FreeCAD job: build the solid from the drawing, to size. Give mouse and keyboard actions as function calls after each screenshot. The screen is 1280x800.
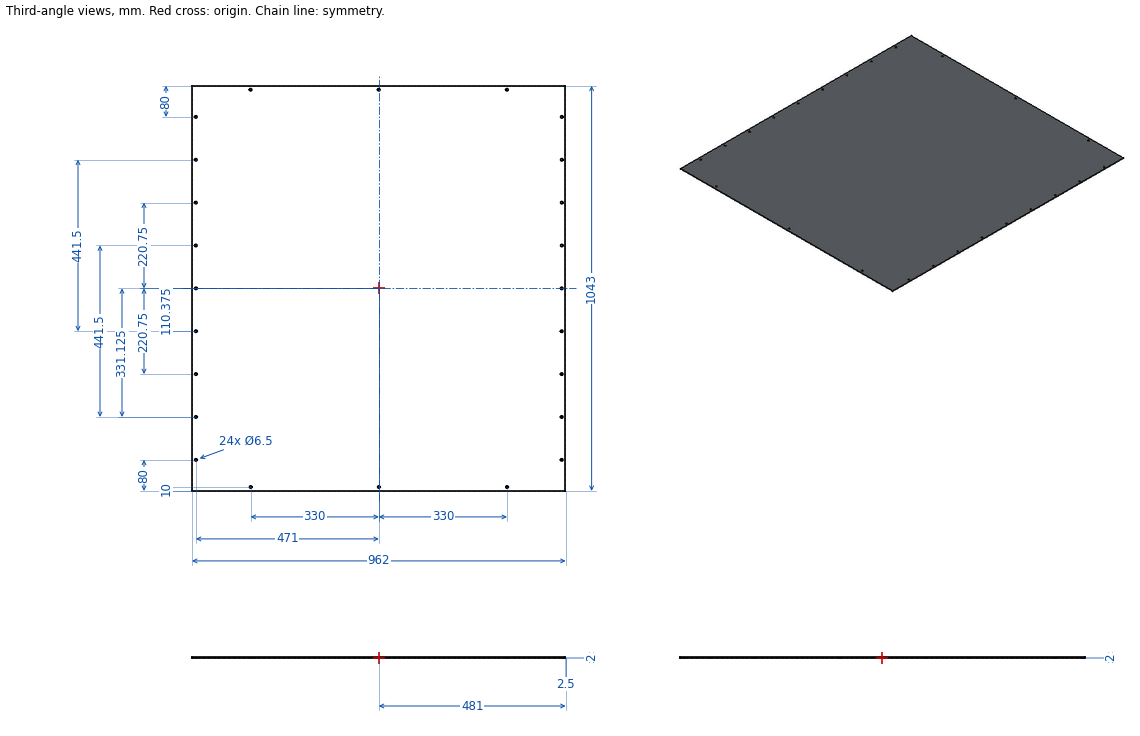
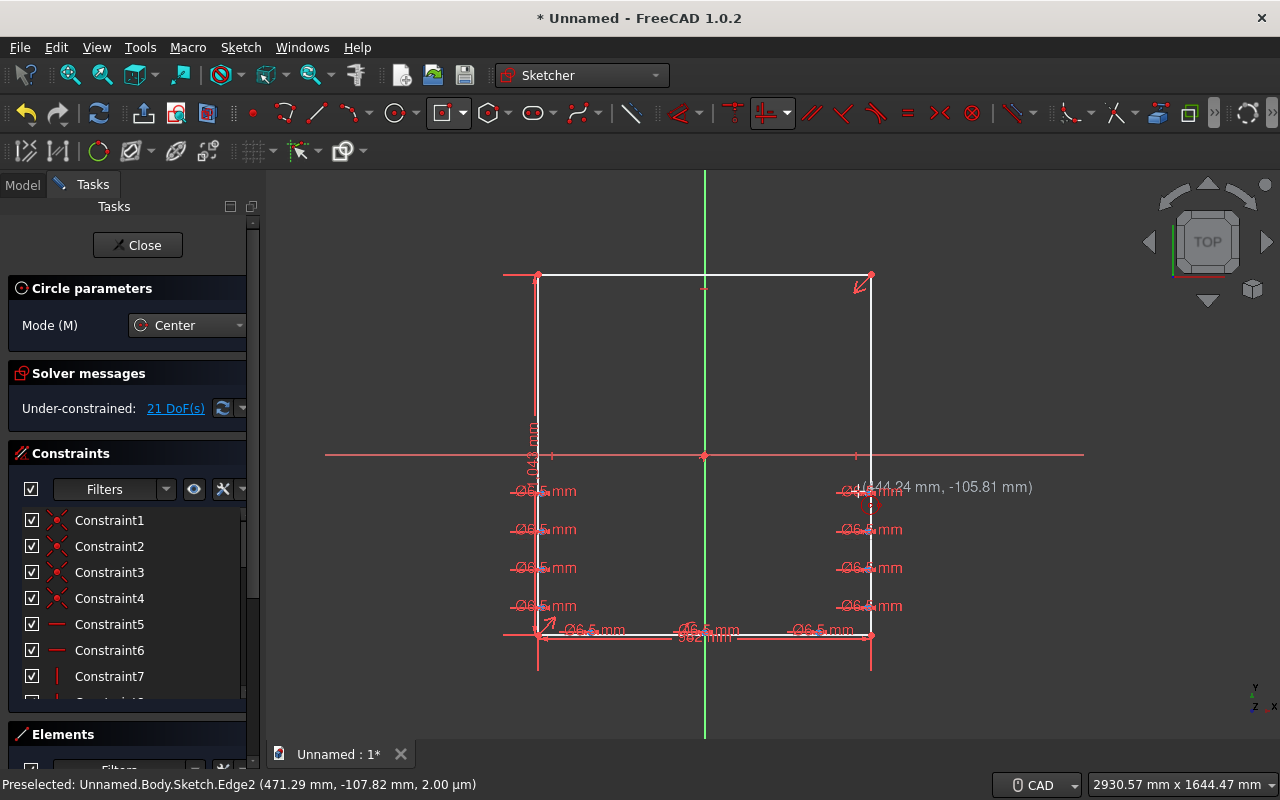
scroll(542, 455, up, 16)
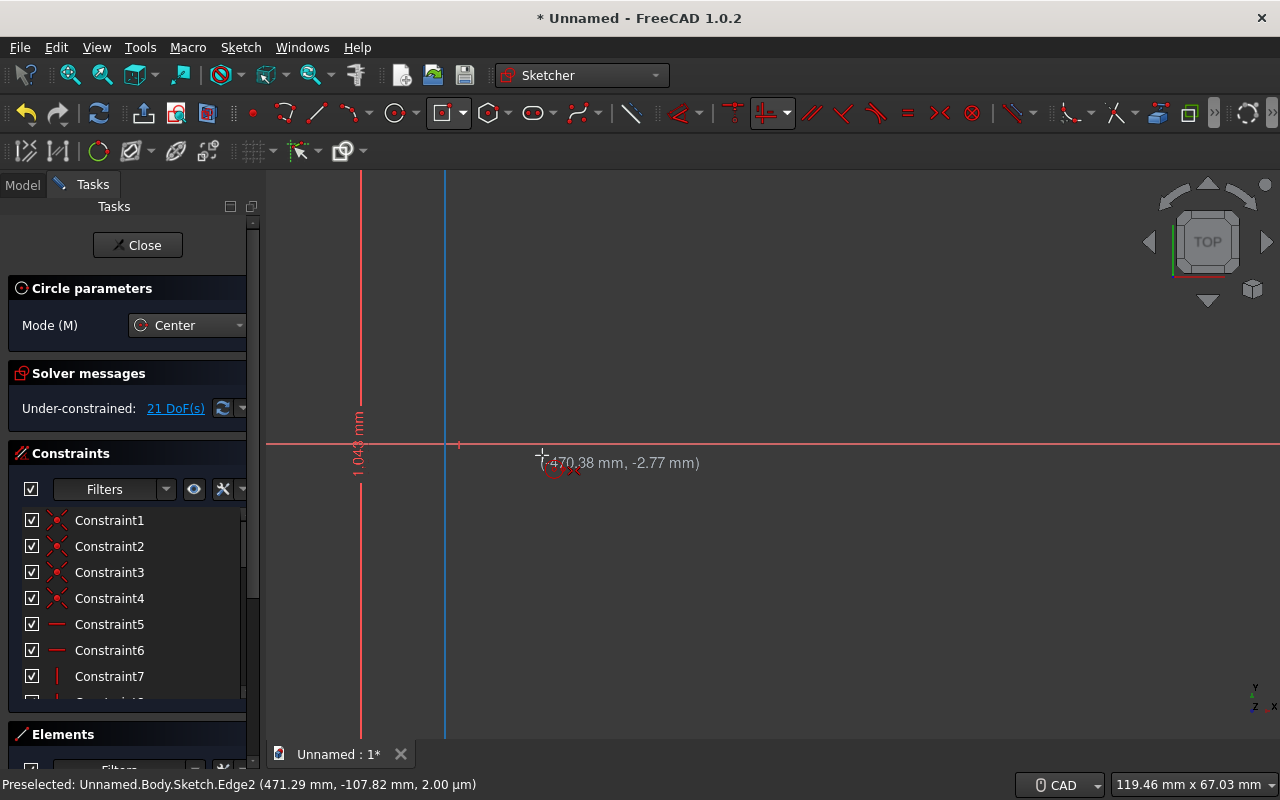
scroll(504, 455, down, 15)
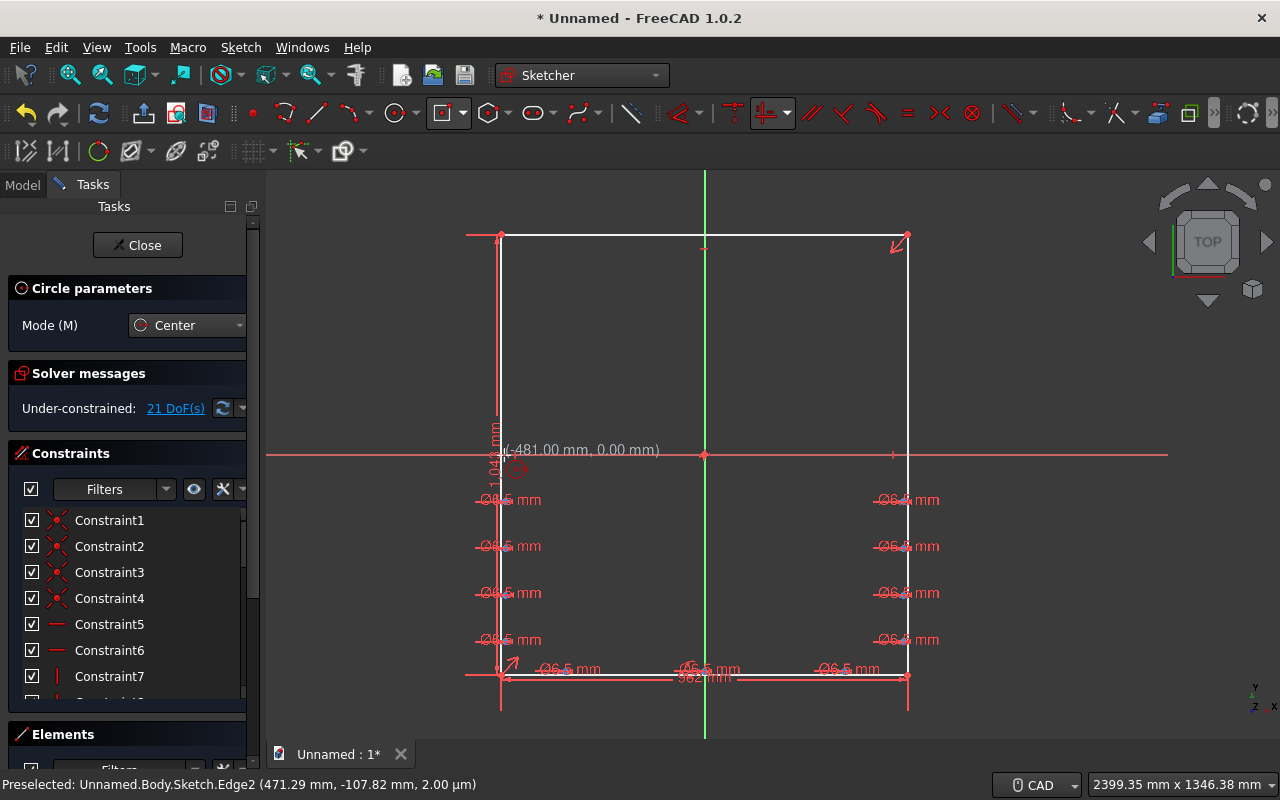
scroll(506, 455, up, 7)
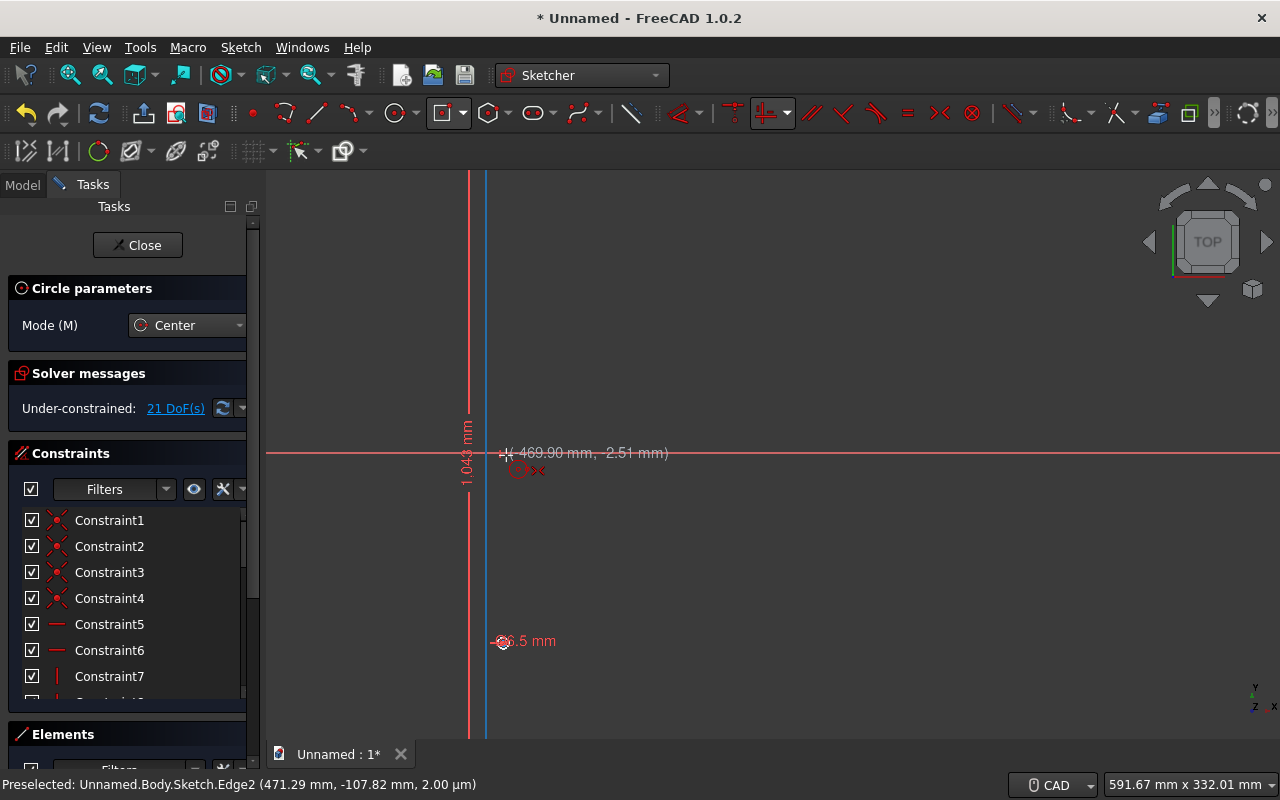
click(503, 453)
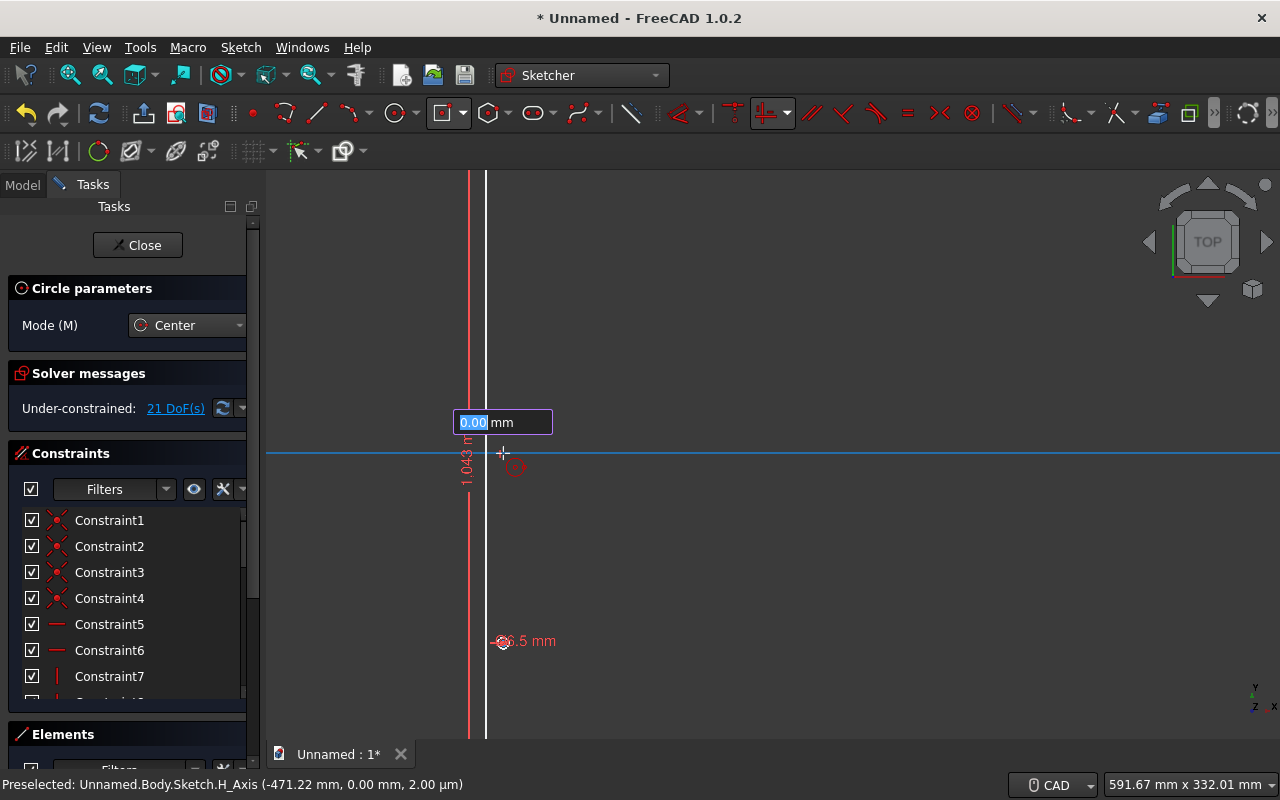
scroll(501, 458, up, 6)
move(502, 458)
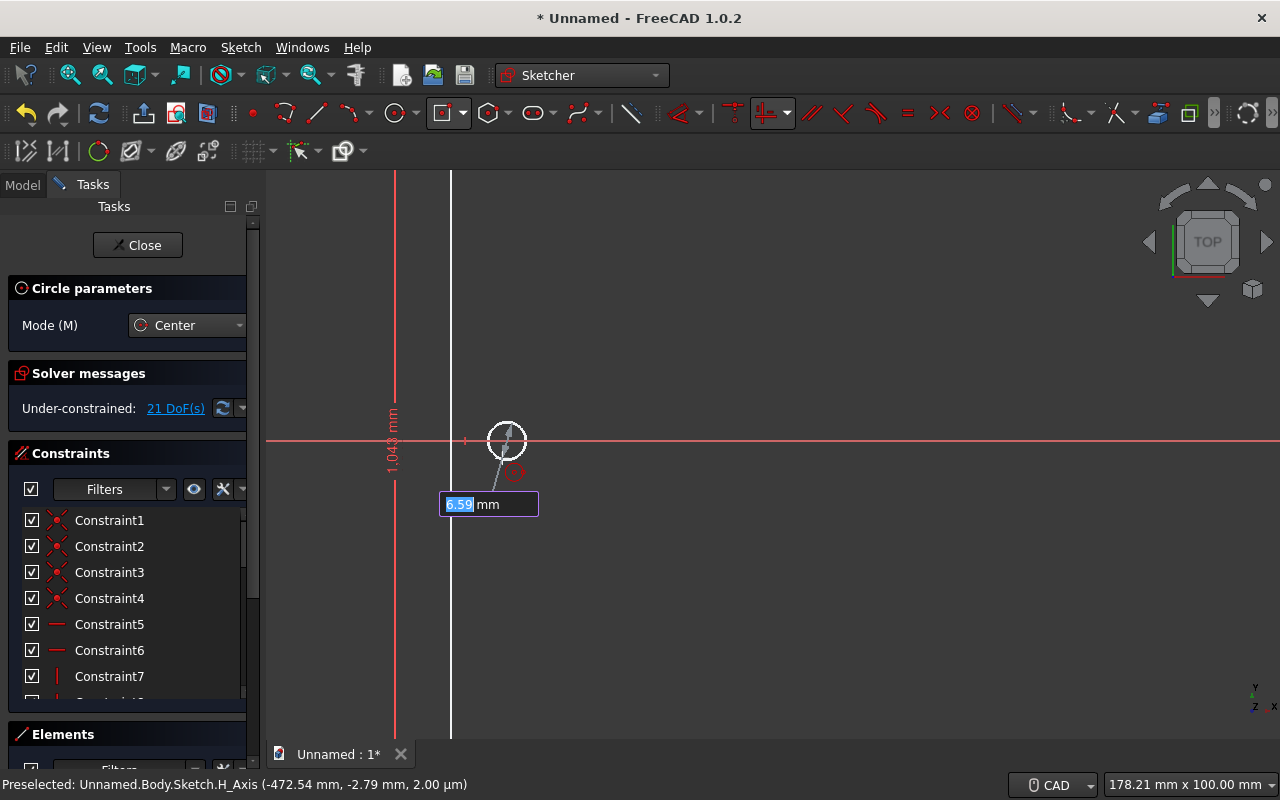
text(6.5)
key(Return)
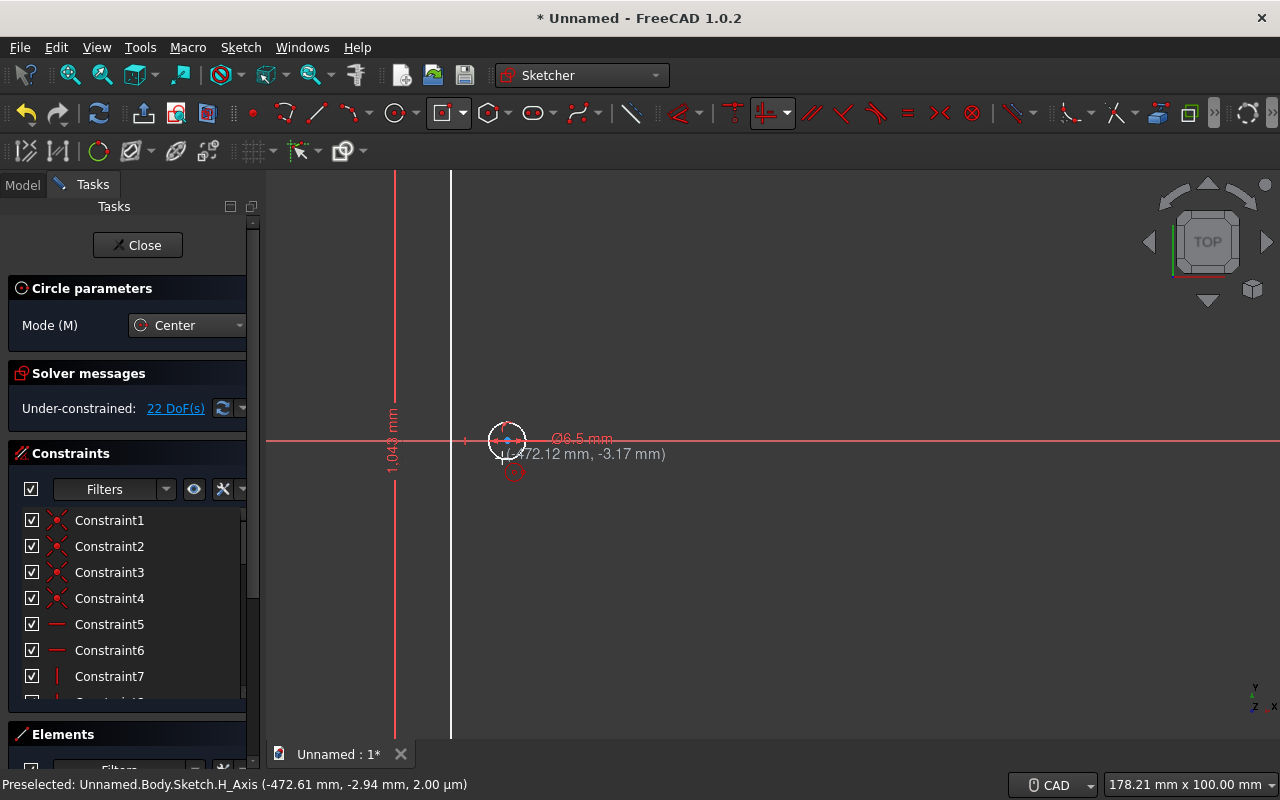
scroll(544, 455, down, 14)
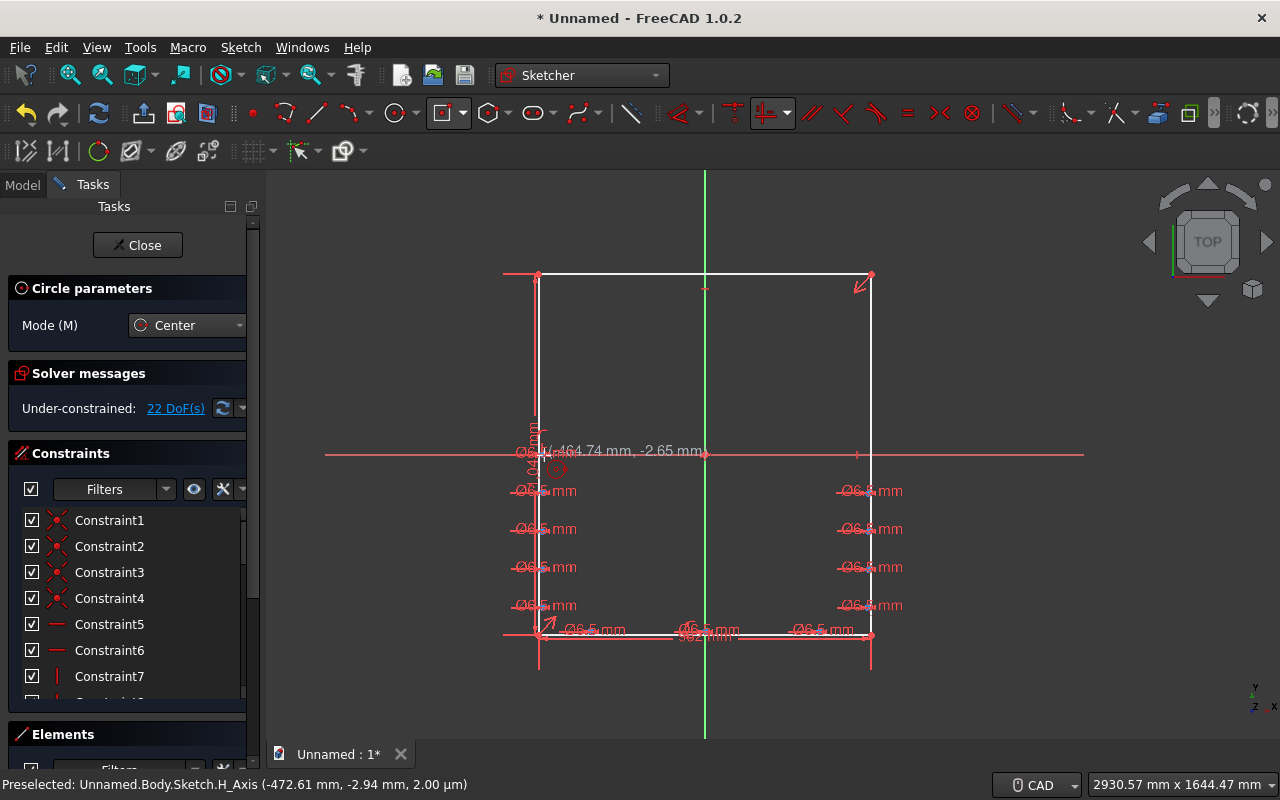
scroll(542, 416, up, 16)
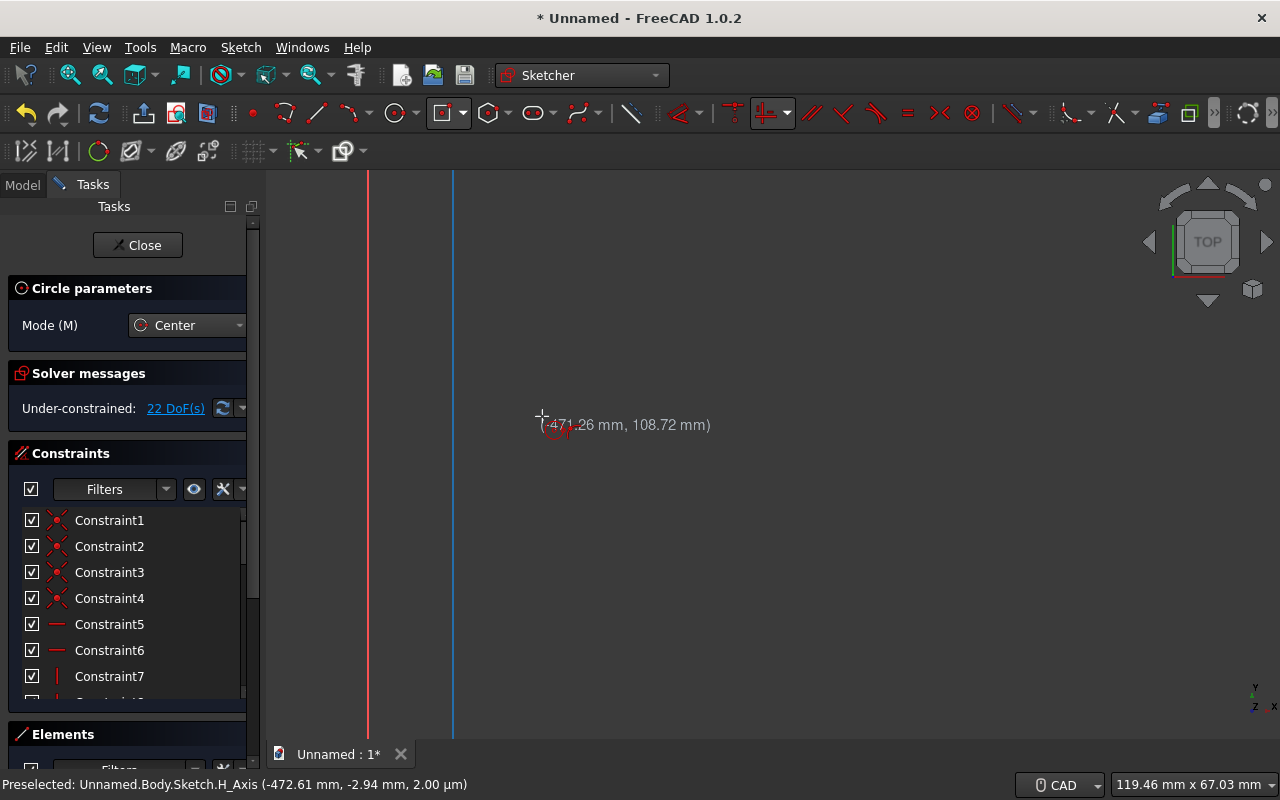
scroll(504, 407, down, 15)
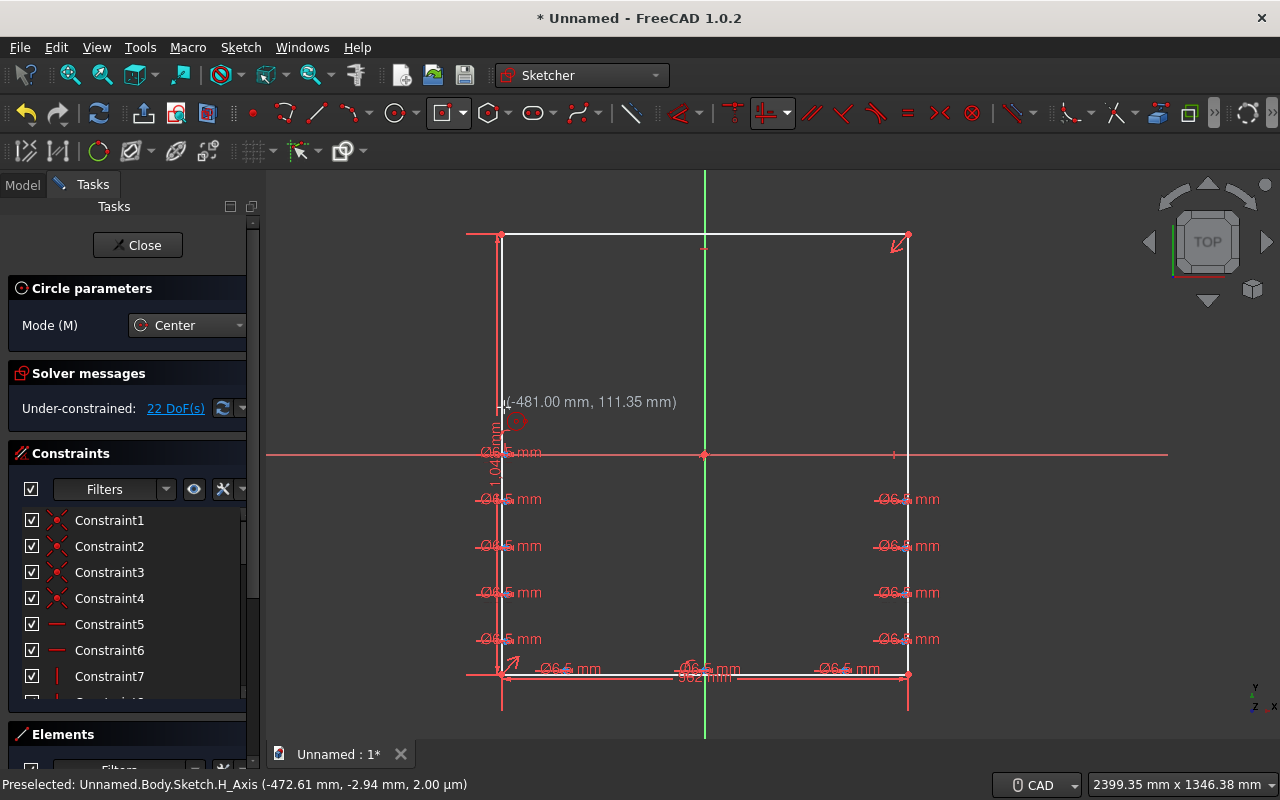
scroll(506, 408, up, 7)